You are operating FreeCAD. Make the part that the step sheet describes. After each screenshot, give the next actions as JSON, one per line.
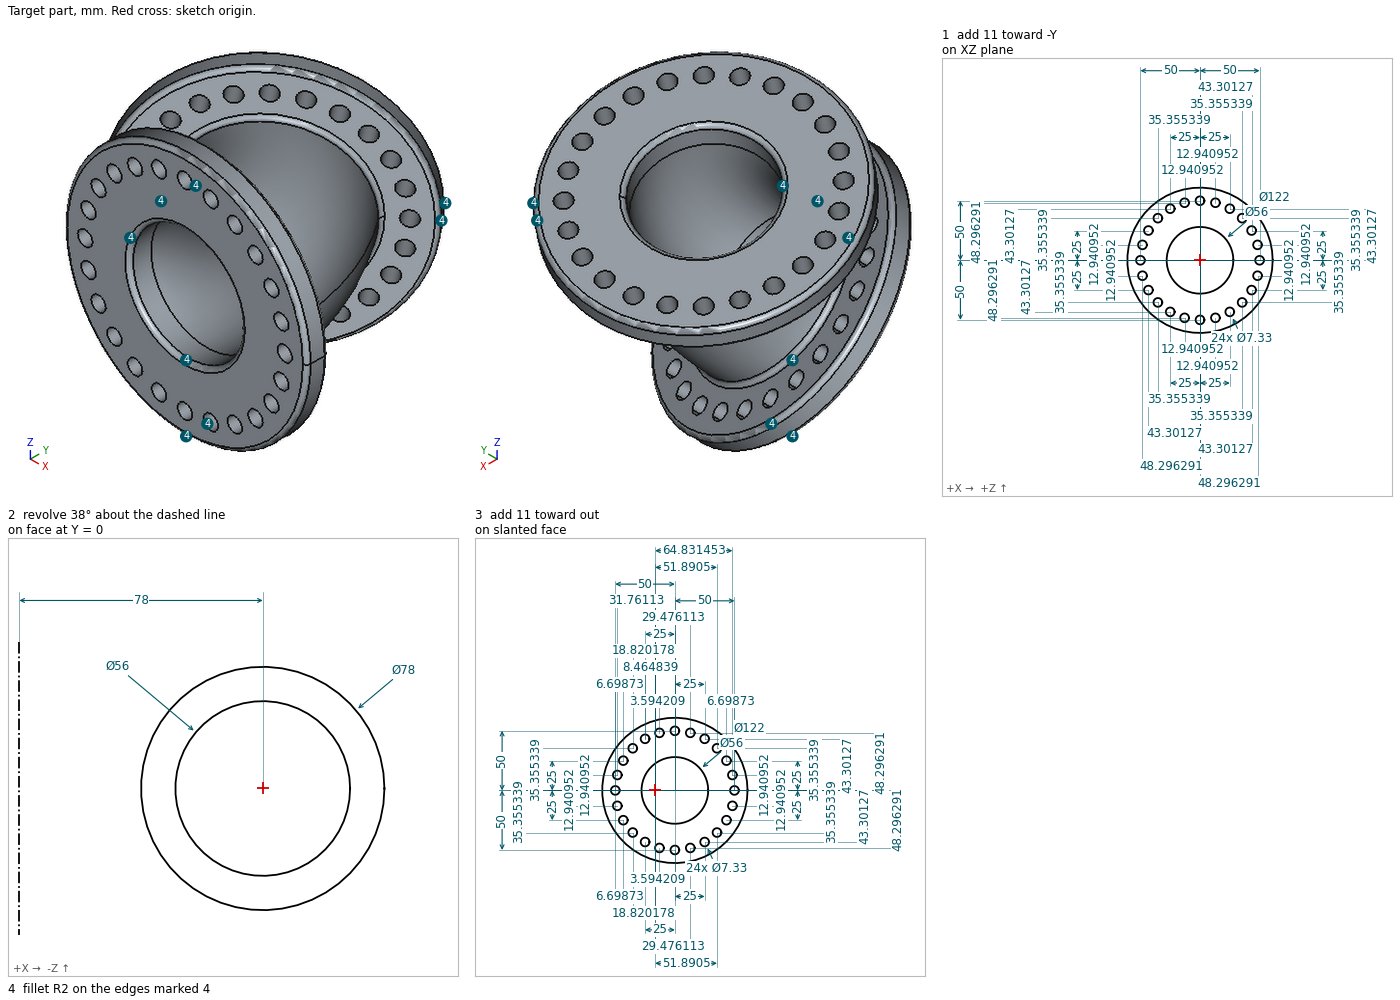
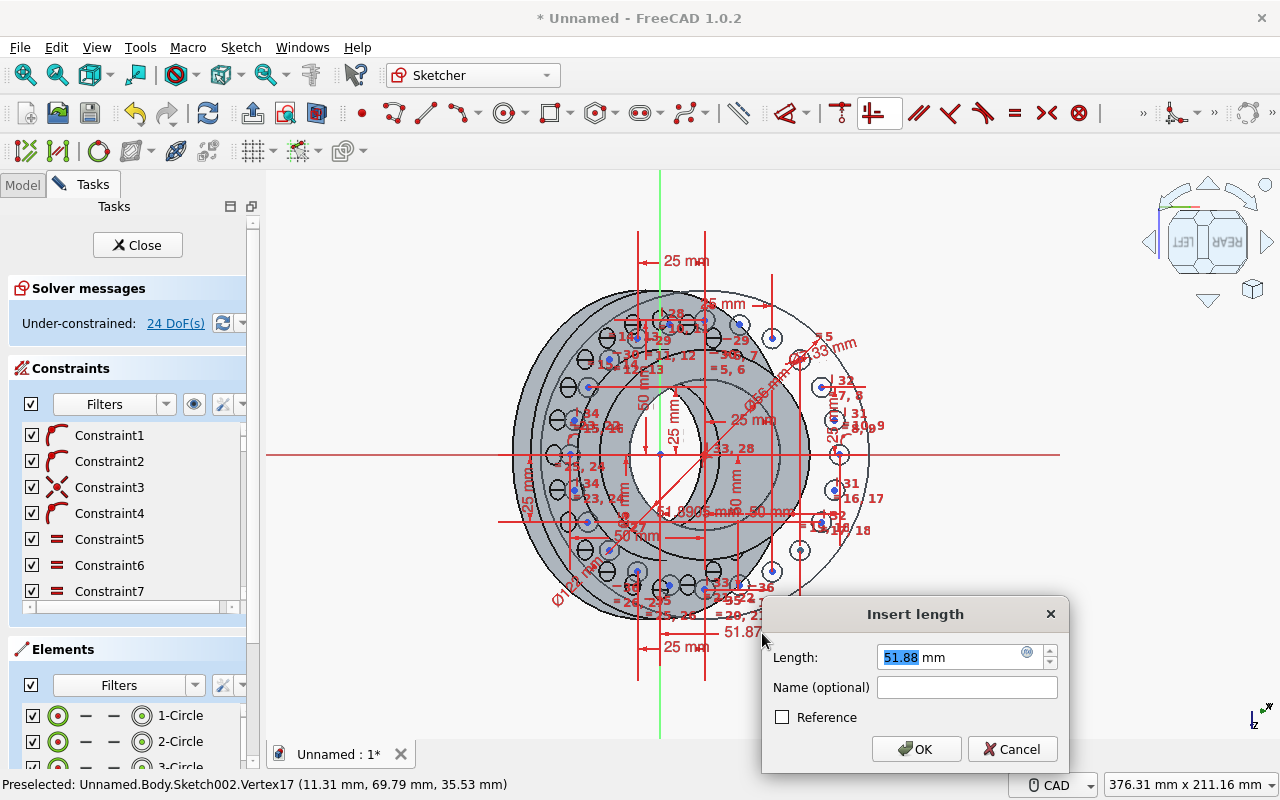
{"action": "type", "text": "51.8905"}
{"action": "key", "text": "Return"}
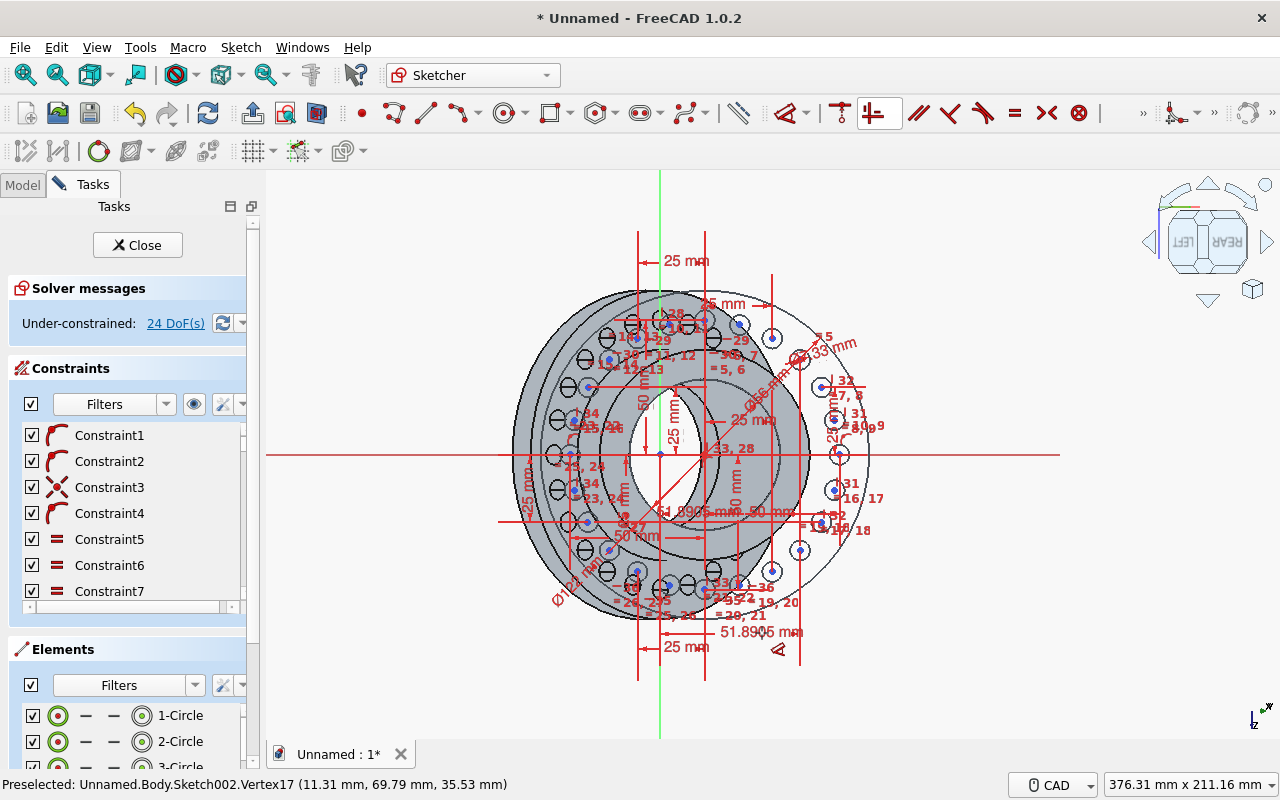
{"action": "left_click", "coordinate": [772, 339]}
{"action": "left_click", "coordinate": [602, 423]}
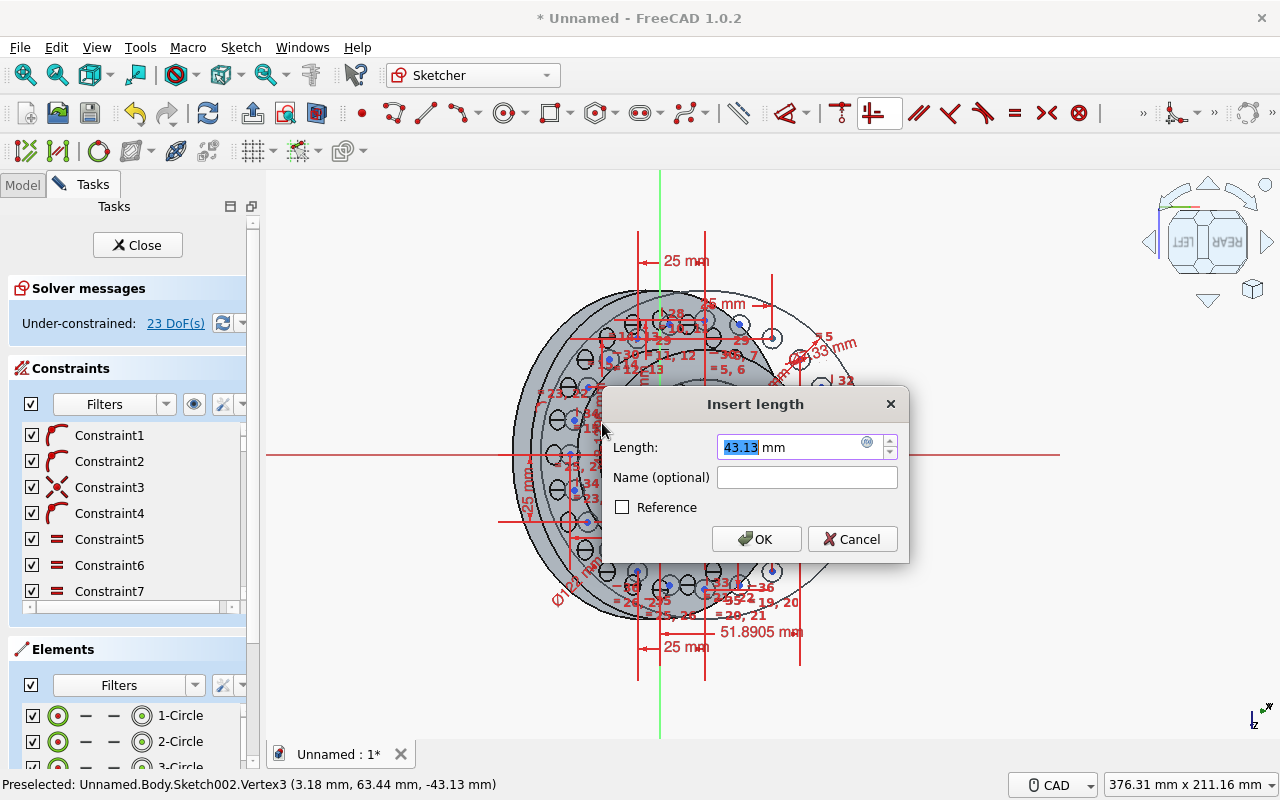
{"action": "type", "text": "43.30127"}
{"action": "key", "text": "Return"}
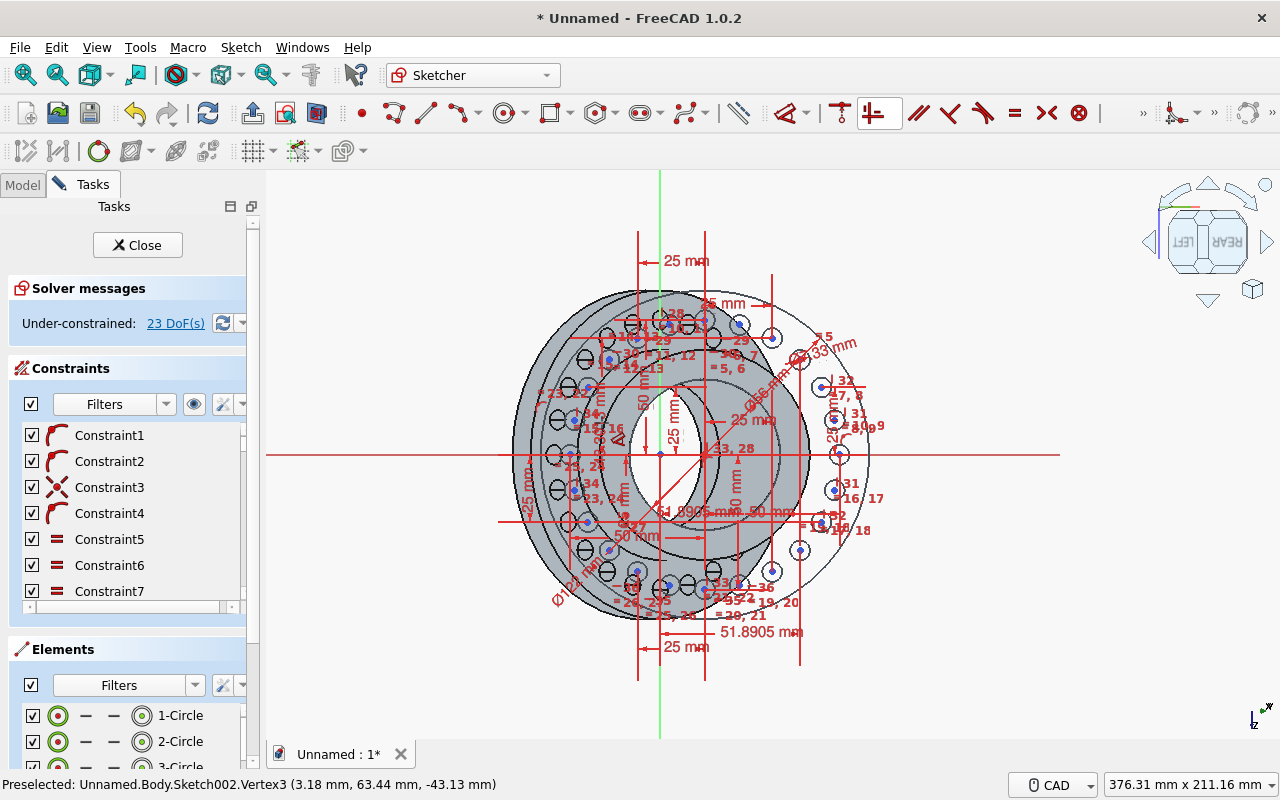
{"action": "scroll", "coordinate": [670, 325], "scroll_direction": "up", "scroll_amount": 8}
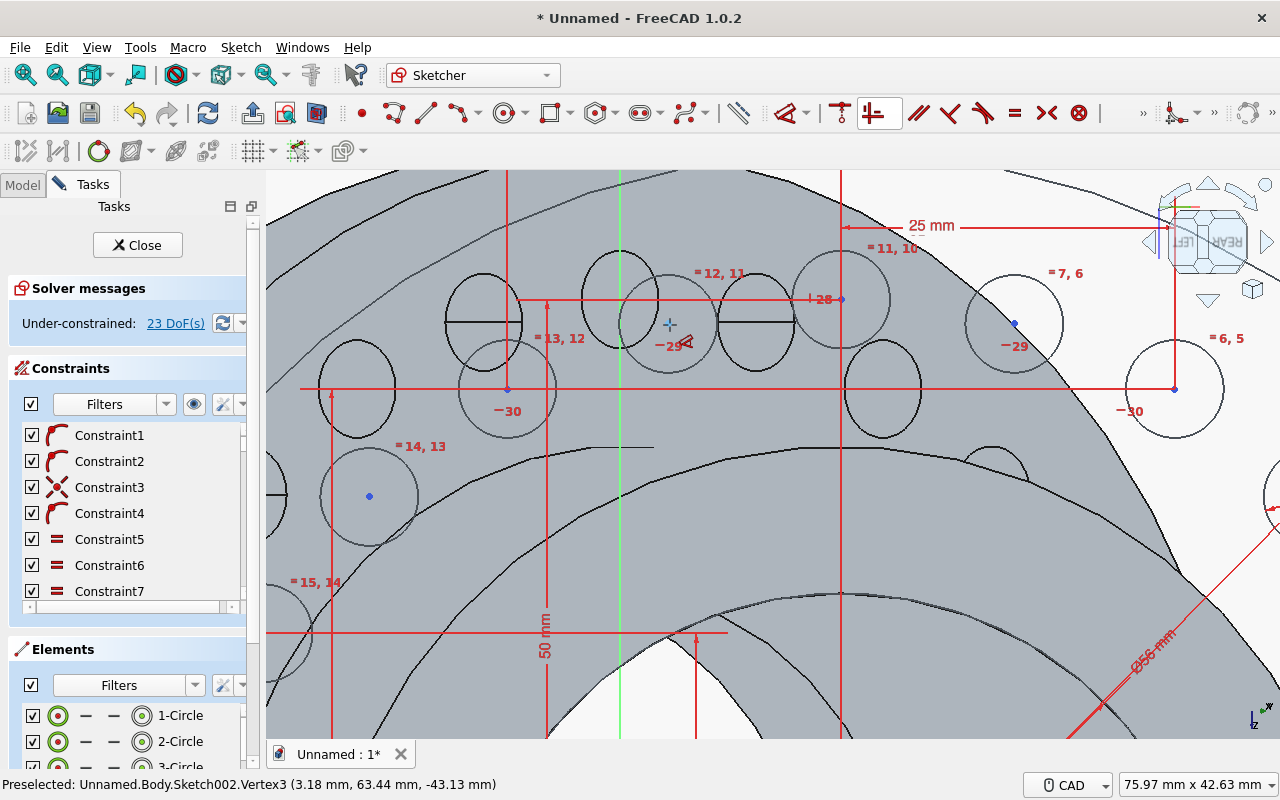
{"action": "left_click", "coordinate": [668, 324]}
{"action": "left_click", "coordinate": [661, 290]}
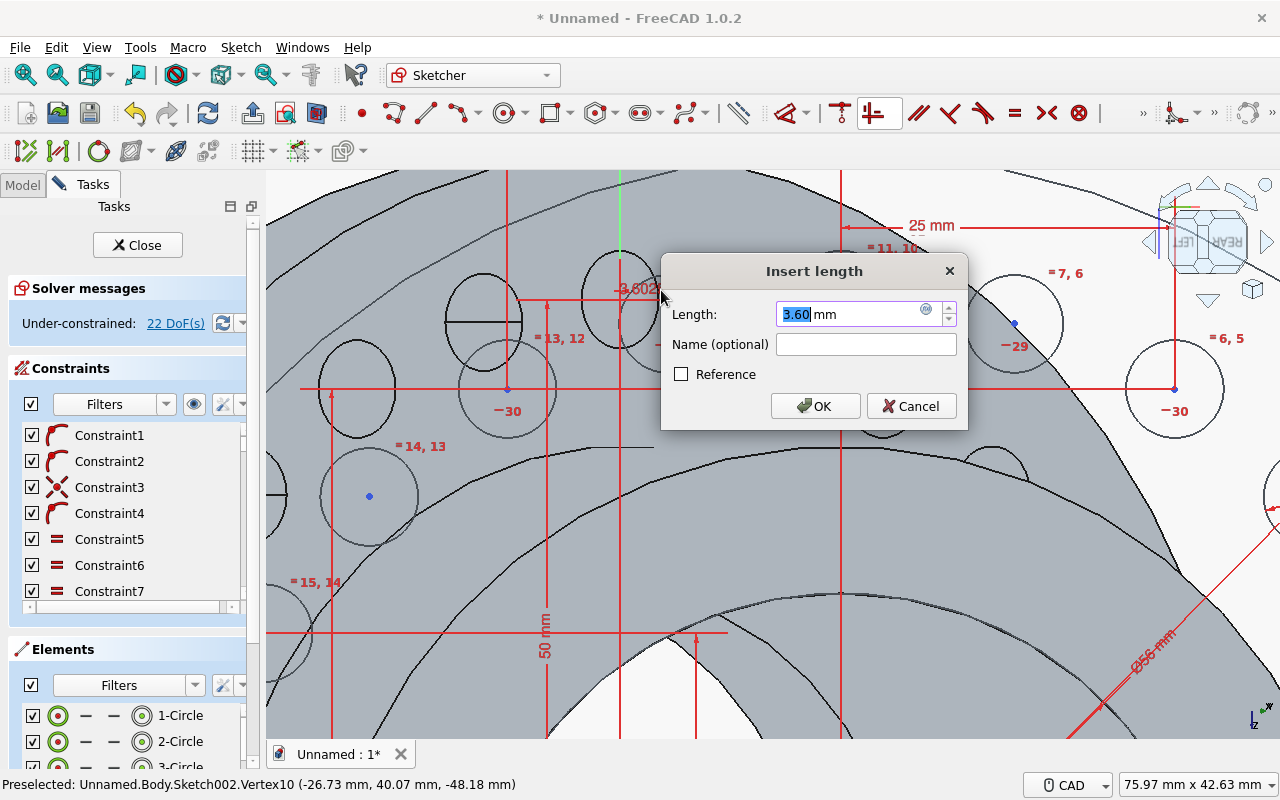
{"action": "type", "text": "3.594209"}
{"action": "key", "text": "Return"}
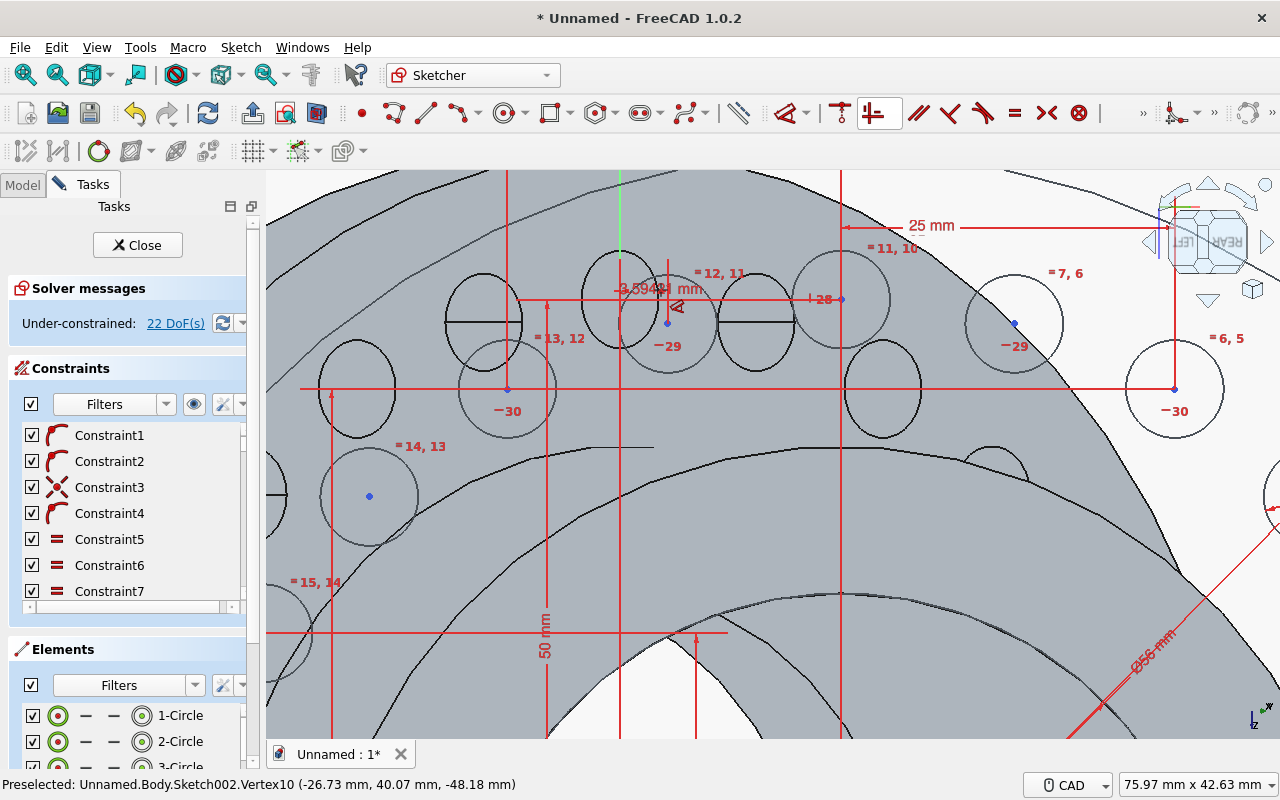
{"action": "left_click", "coordinate": [507, 389]}
{"action": "left_click", "coordinate": [564, 355]}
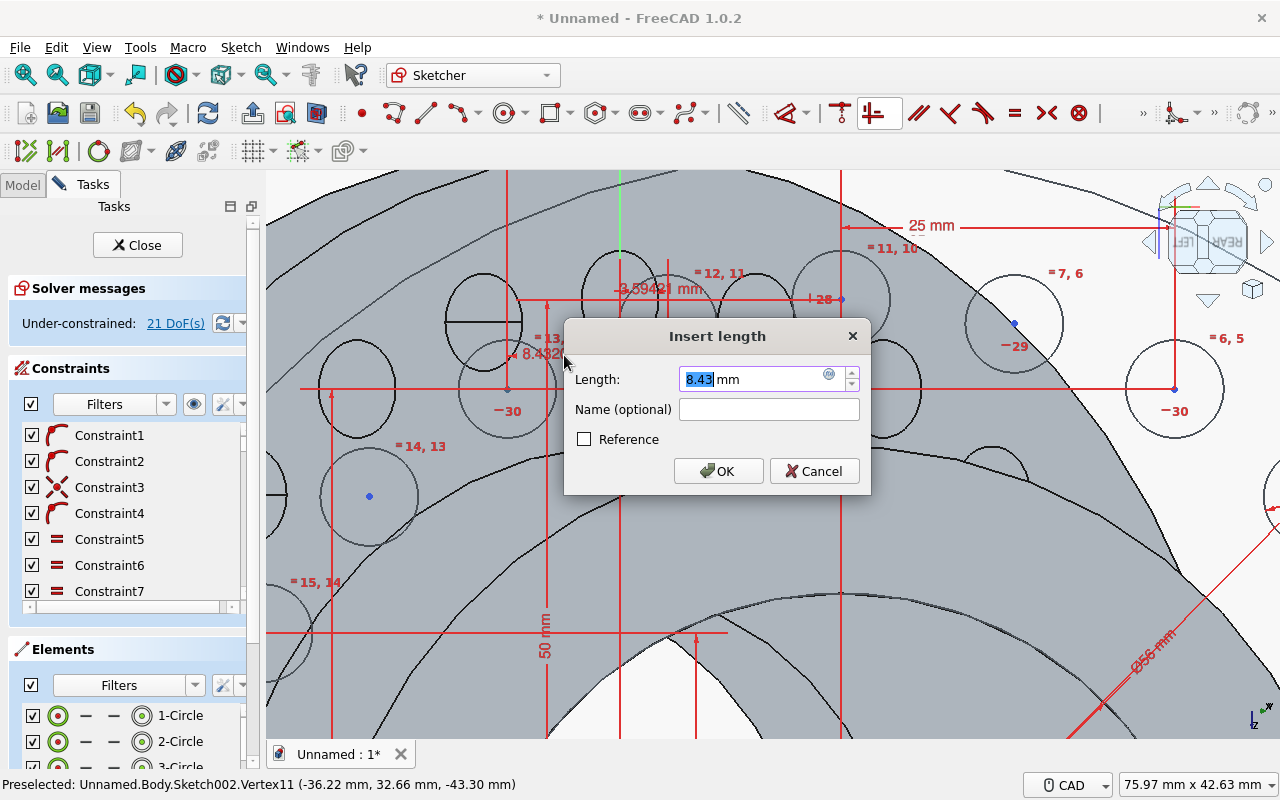
{"action": "type", "text": "8.464839"}
{"action": "key", "text": "Return"}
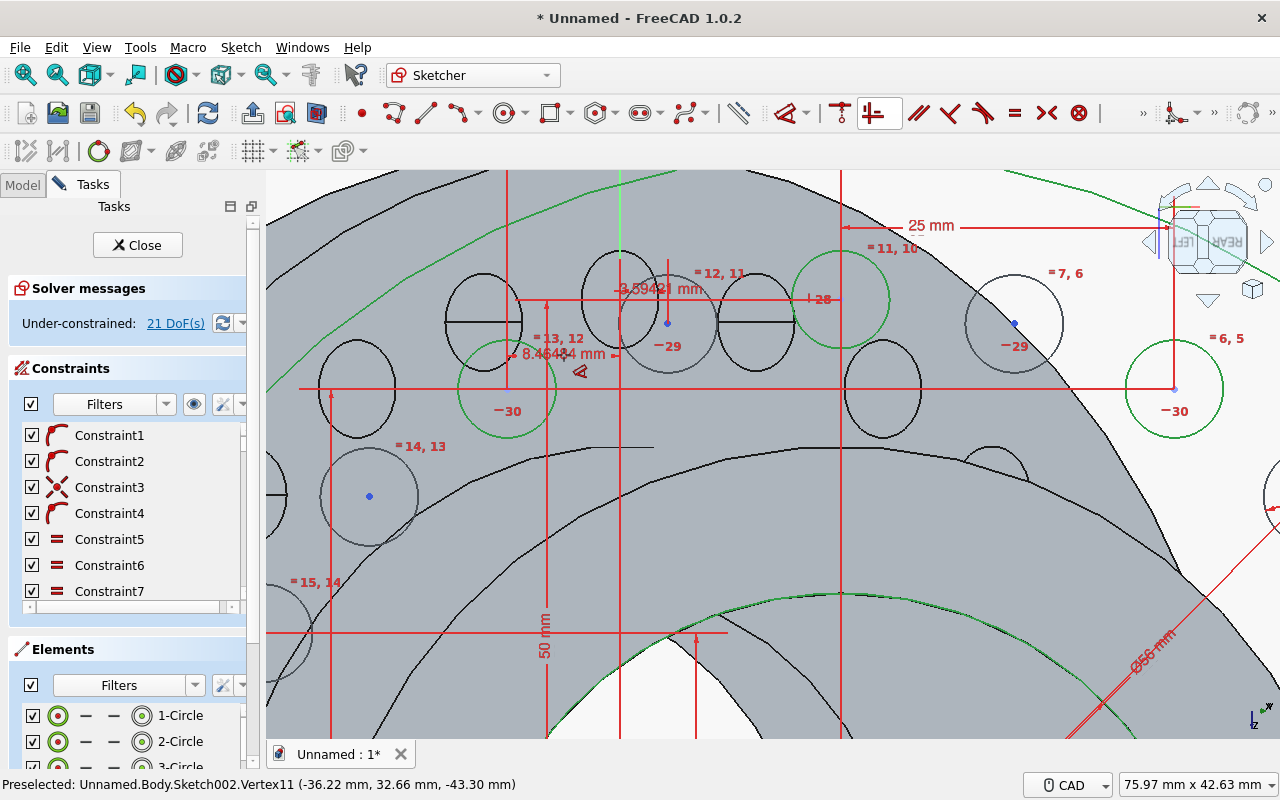
{"action": "scroll", "coordinate": [670, 325], "scroll_direction": "down", "scroll_amount": 8}